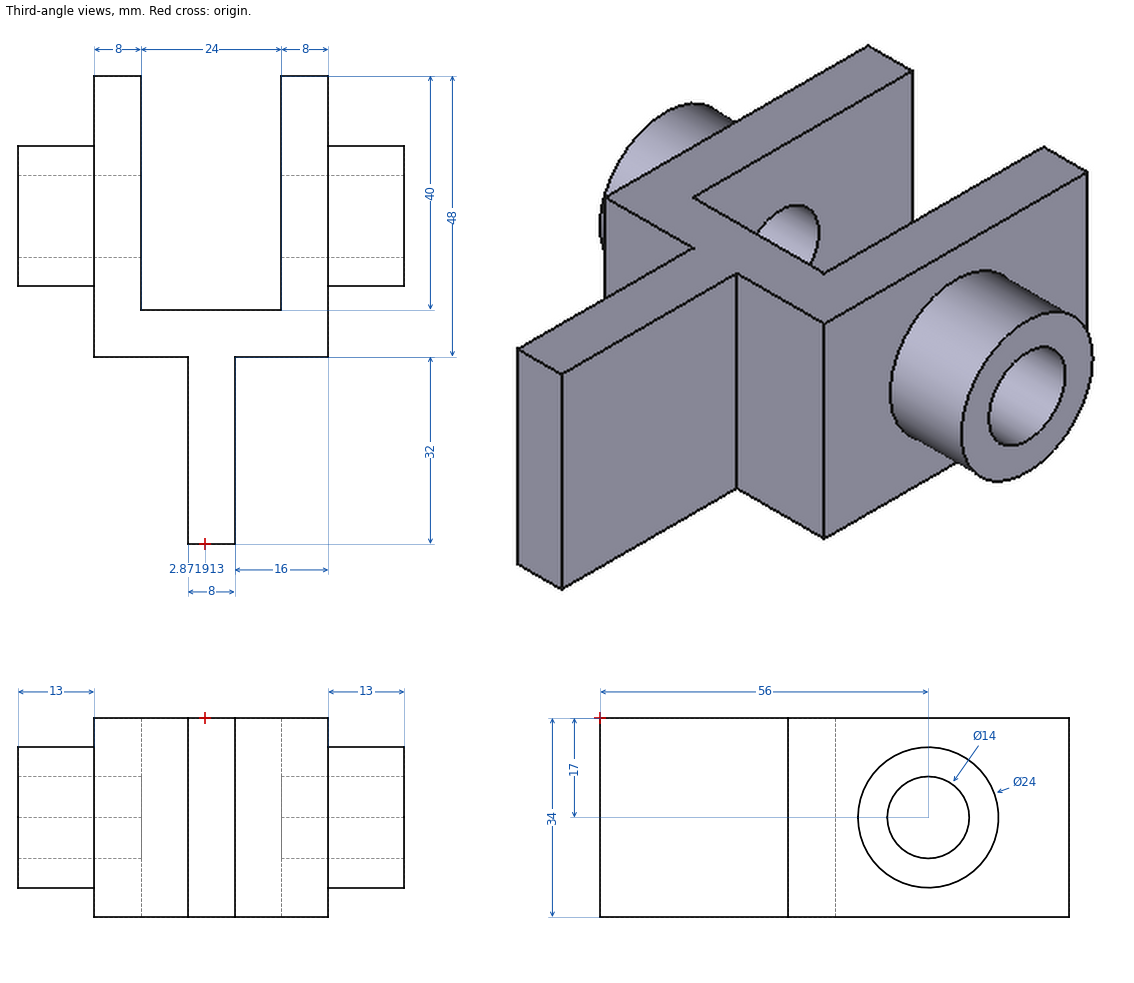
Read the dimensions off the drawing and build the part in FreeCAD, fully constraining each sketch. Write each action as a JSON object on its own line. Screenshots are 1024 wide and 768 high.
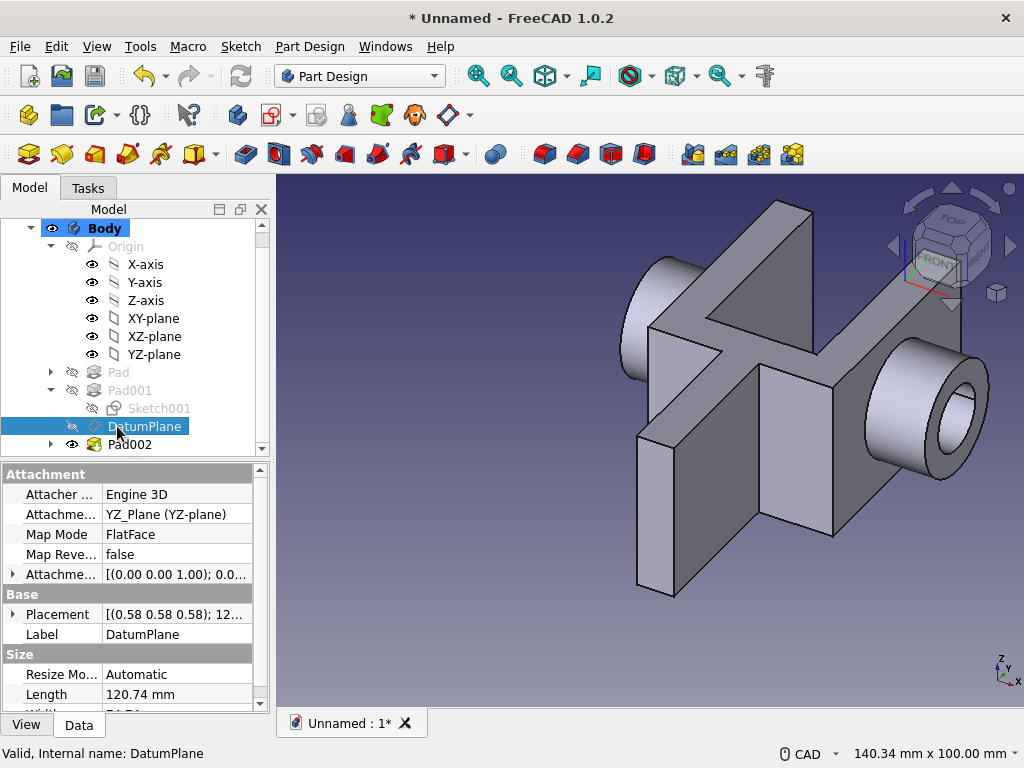
{"action": "key", "text": "6"}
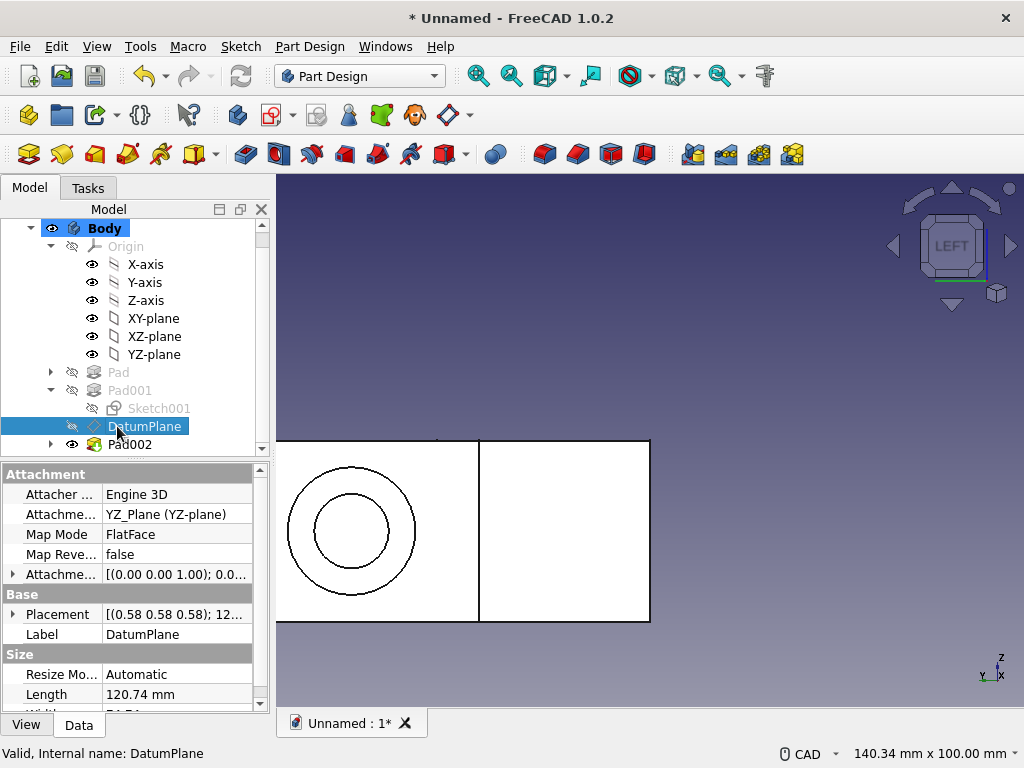
{"action": "left_click", "coordinate": [479, 76]}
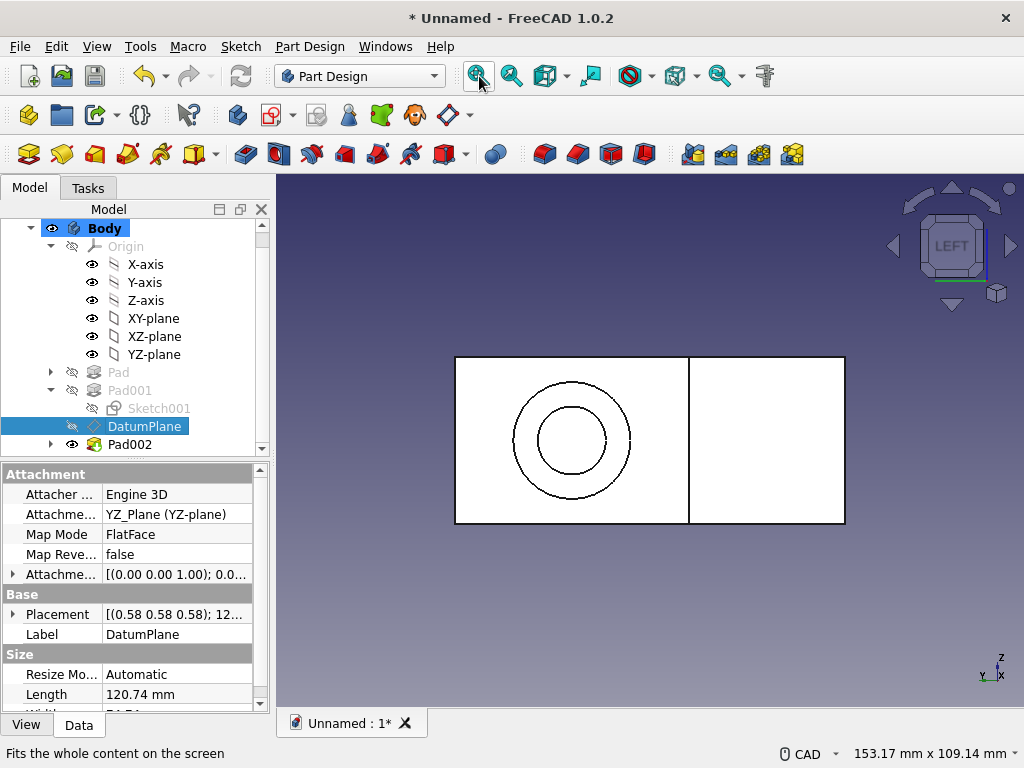
{"action": "left_click", "coordinate": [639, 392]}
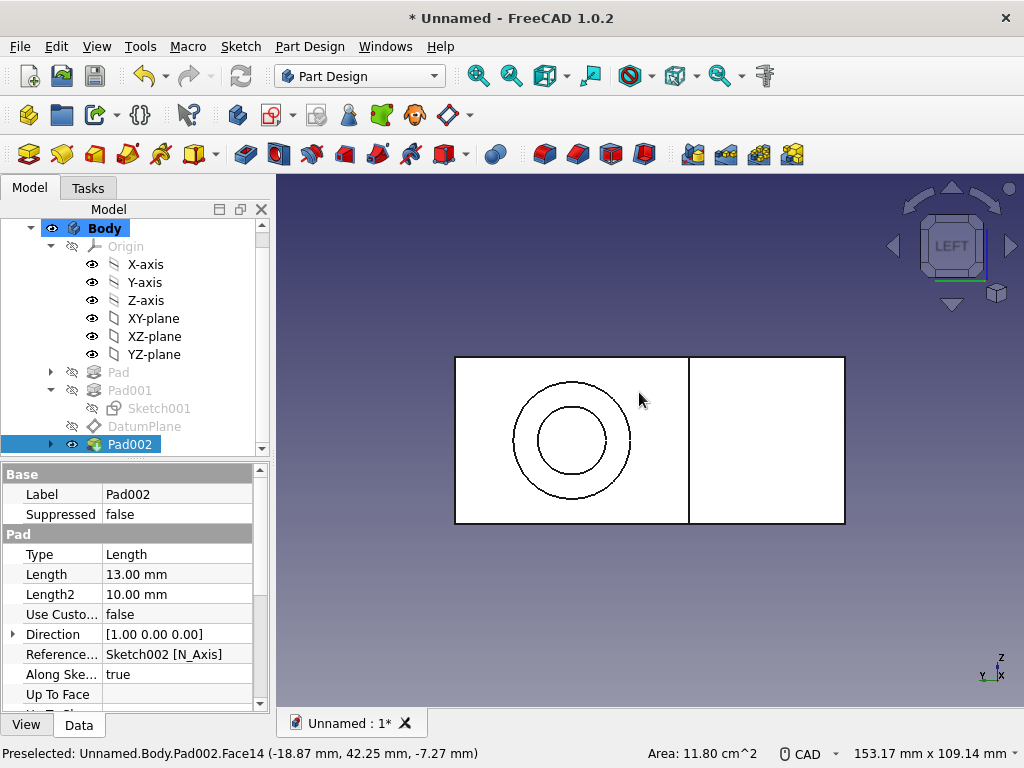
{"action": "left_click", "coordinate": [270, 116]}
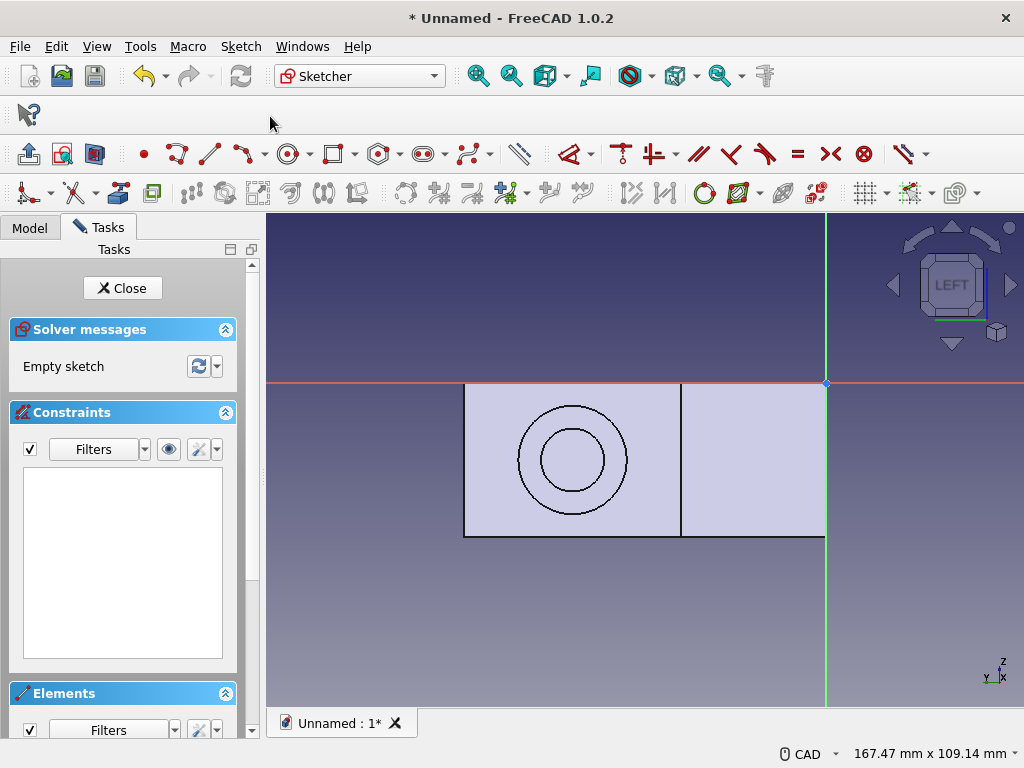
{"action": "key", "text": "q s"}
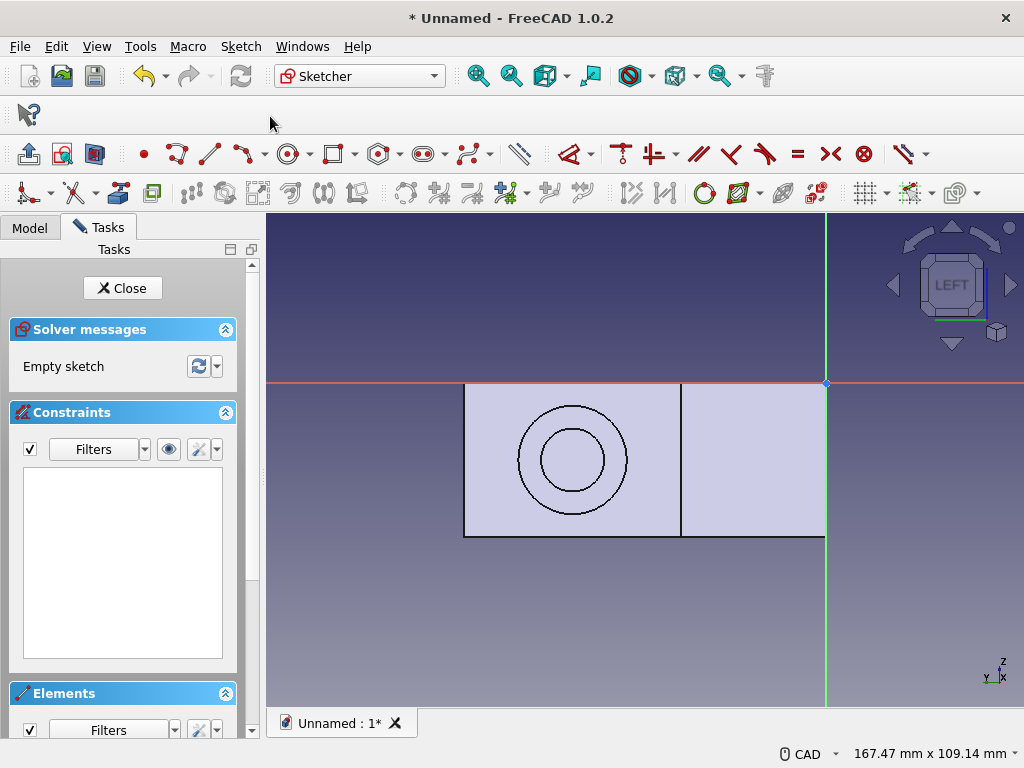
{"action": "scroll", "coordinate": [572, 460], "scroll_direction": "up", "scroll_amount": 8}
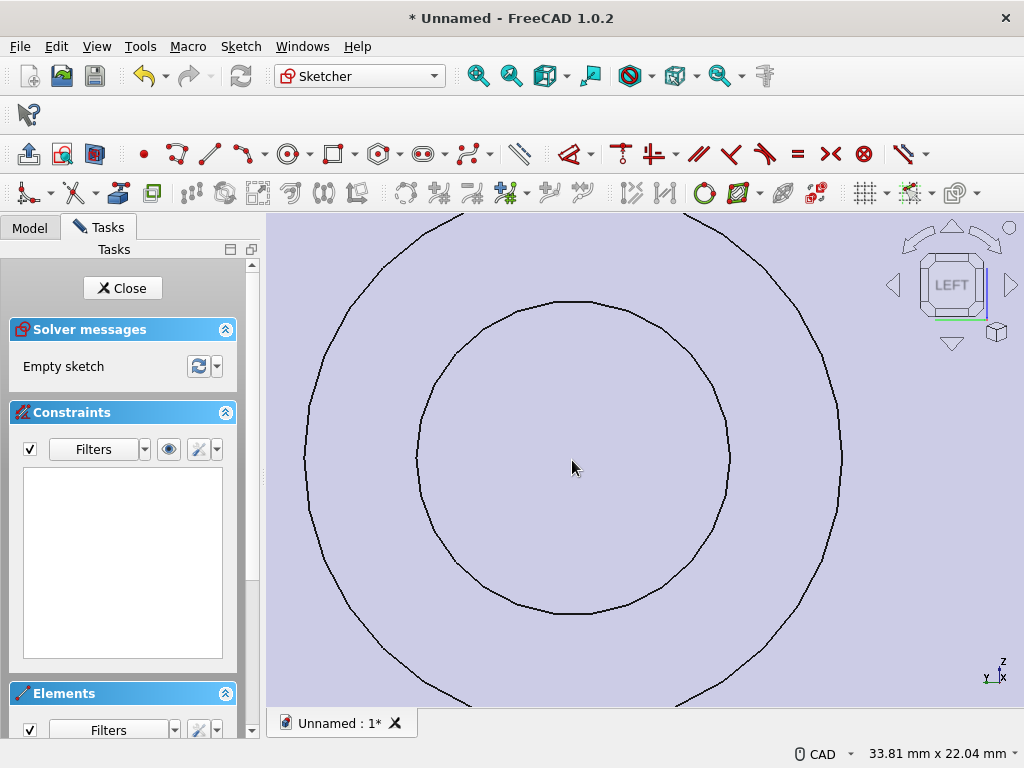
{"action": "key", "text": "g c"}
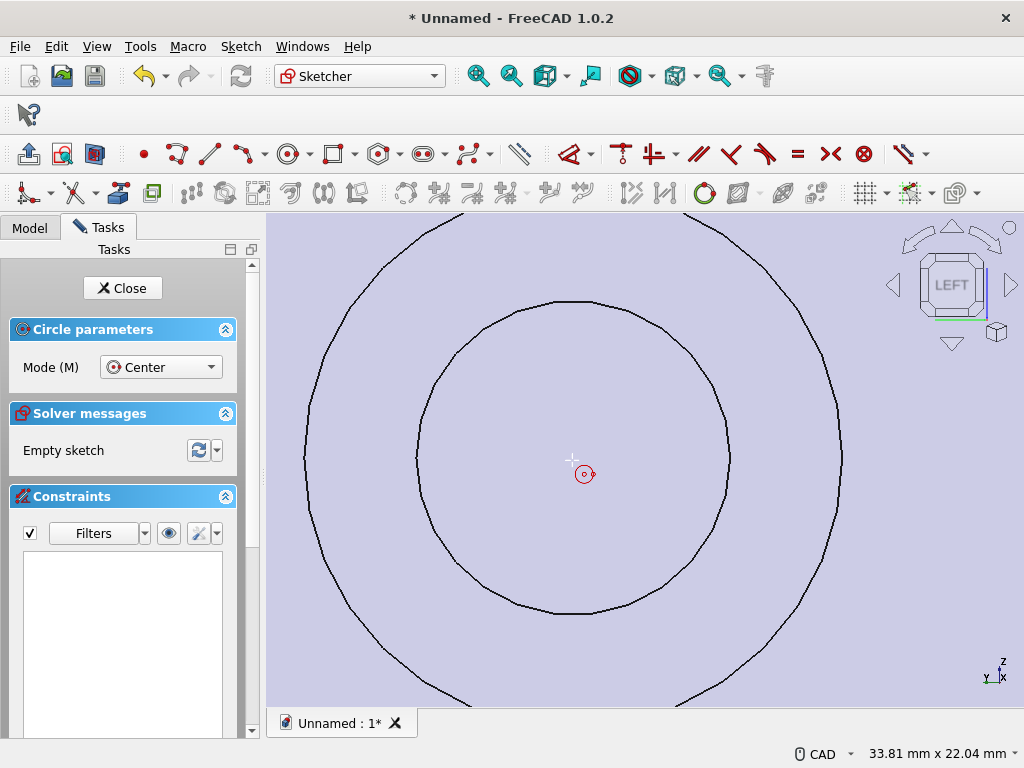
{"action": "left_click", "coordinate": [573, 458]}
{"action": "mouse_move", "coordinate": [684, 347]}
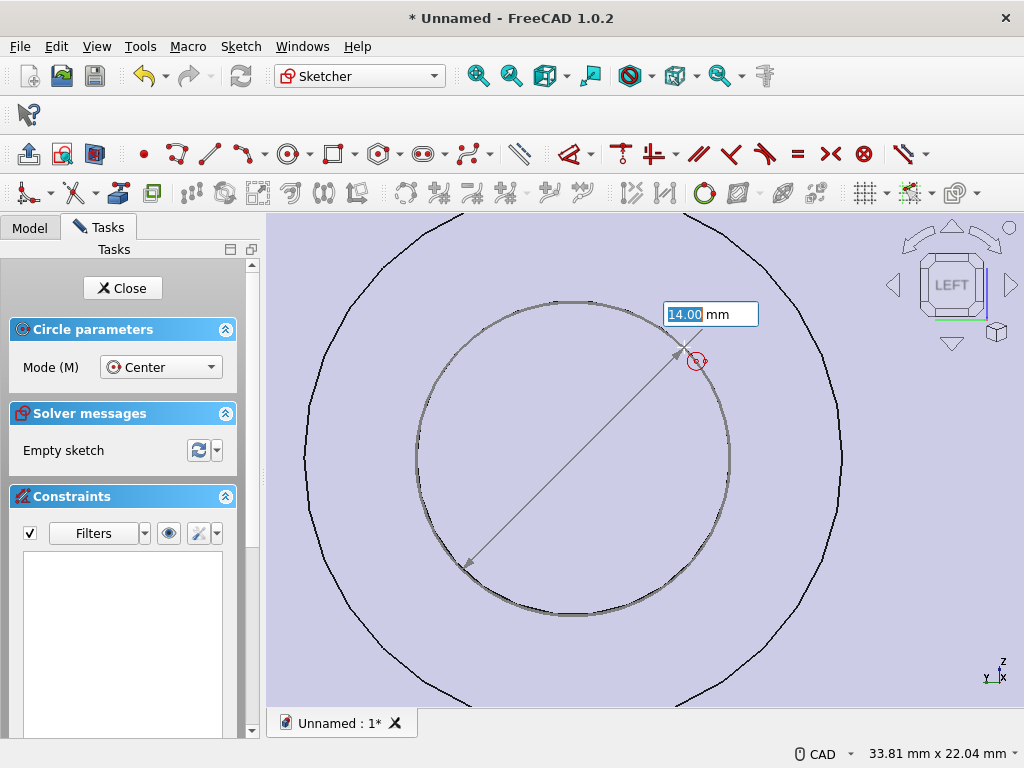
{"action": "type", "text": "14"}
{"action": "key", "text": "Return"}
{"action": "key", "text": "Escape"}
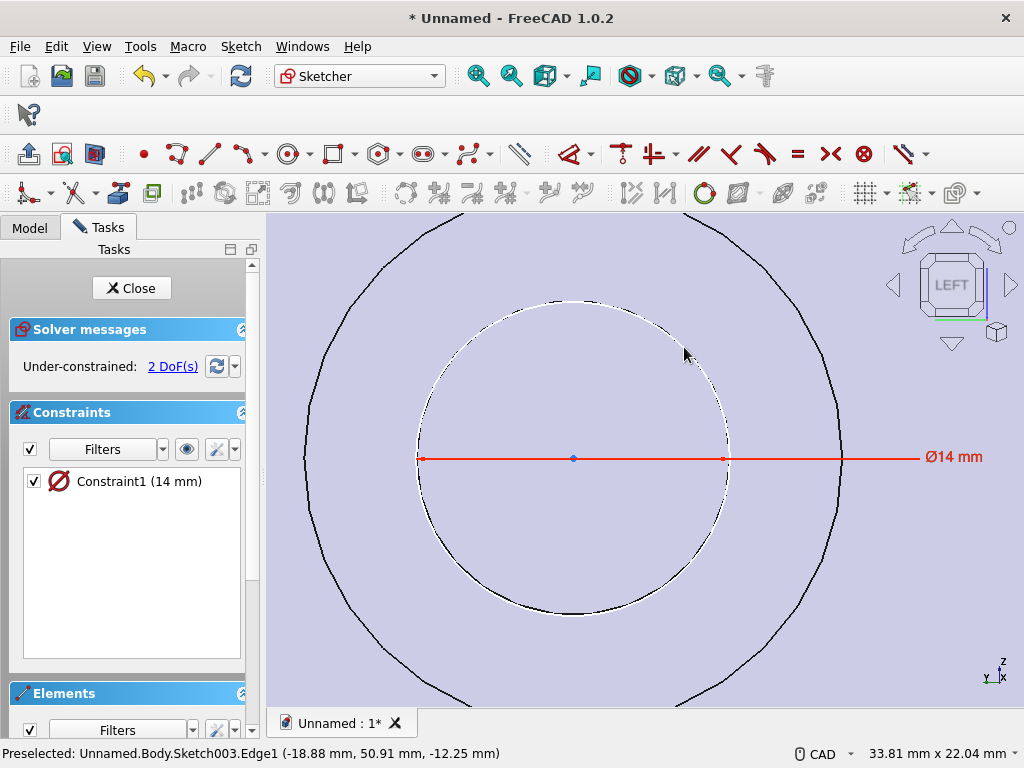
{"action": "key", "text": "d"}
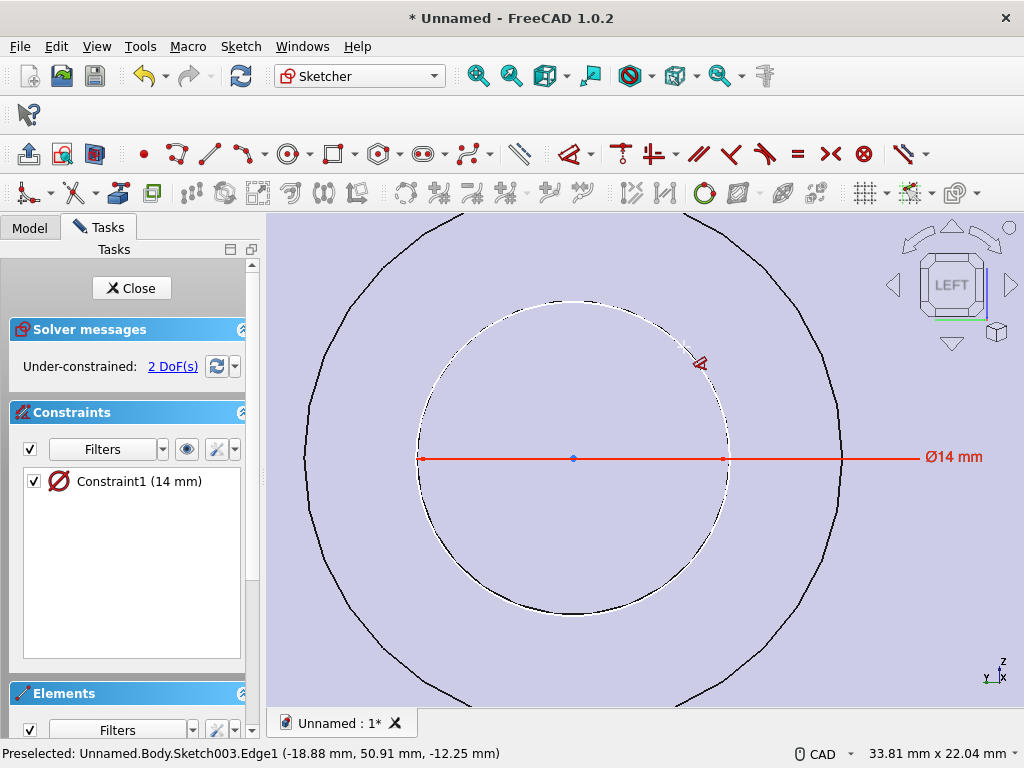
{"action": "left_click", "coordinate": [573, 459]}
{"action": "left_click", "coordinate": [650, 493]}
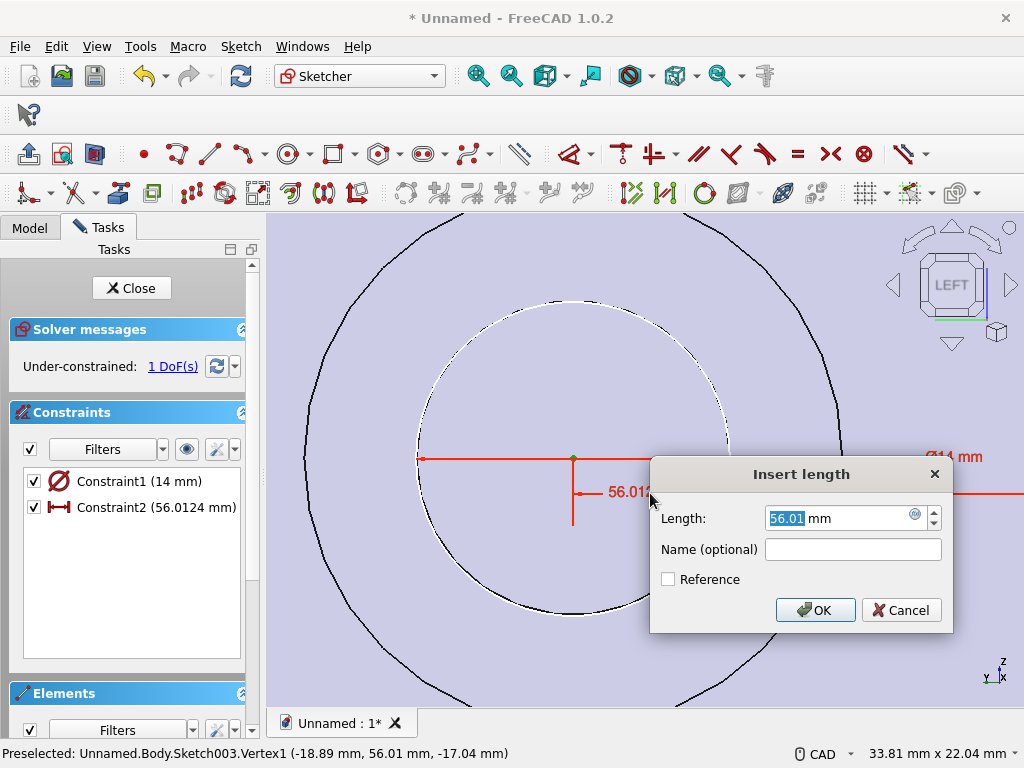
{"action": "type", "text": "56"}
{"action": "key", "text": "Return"}